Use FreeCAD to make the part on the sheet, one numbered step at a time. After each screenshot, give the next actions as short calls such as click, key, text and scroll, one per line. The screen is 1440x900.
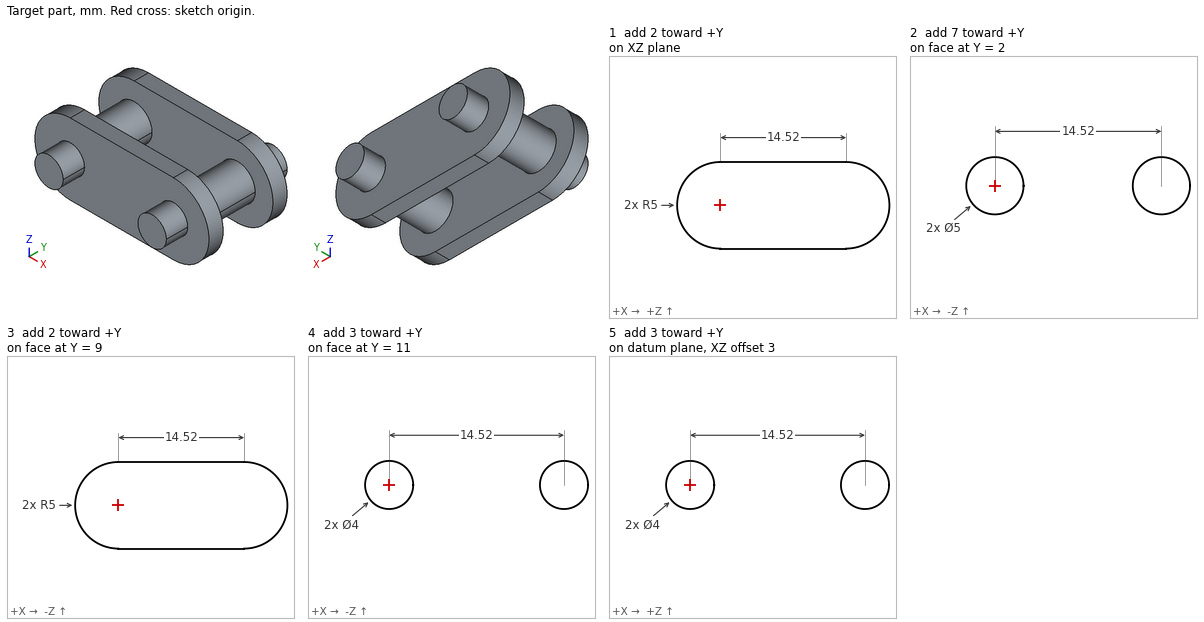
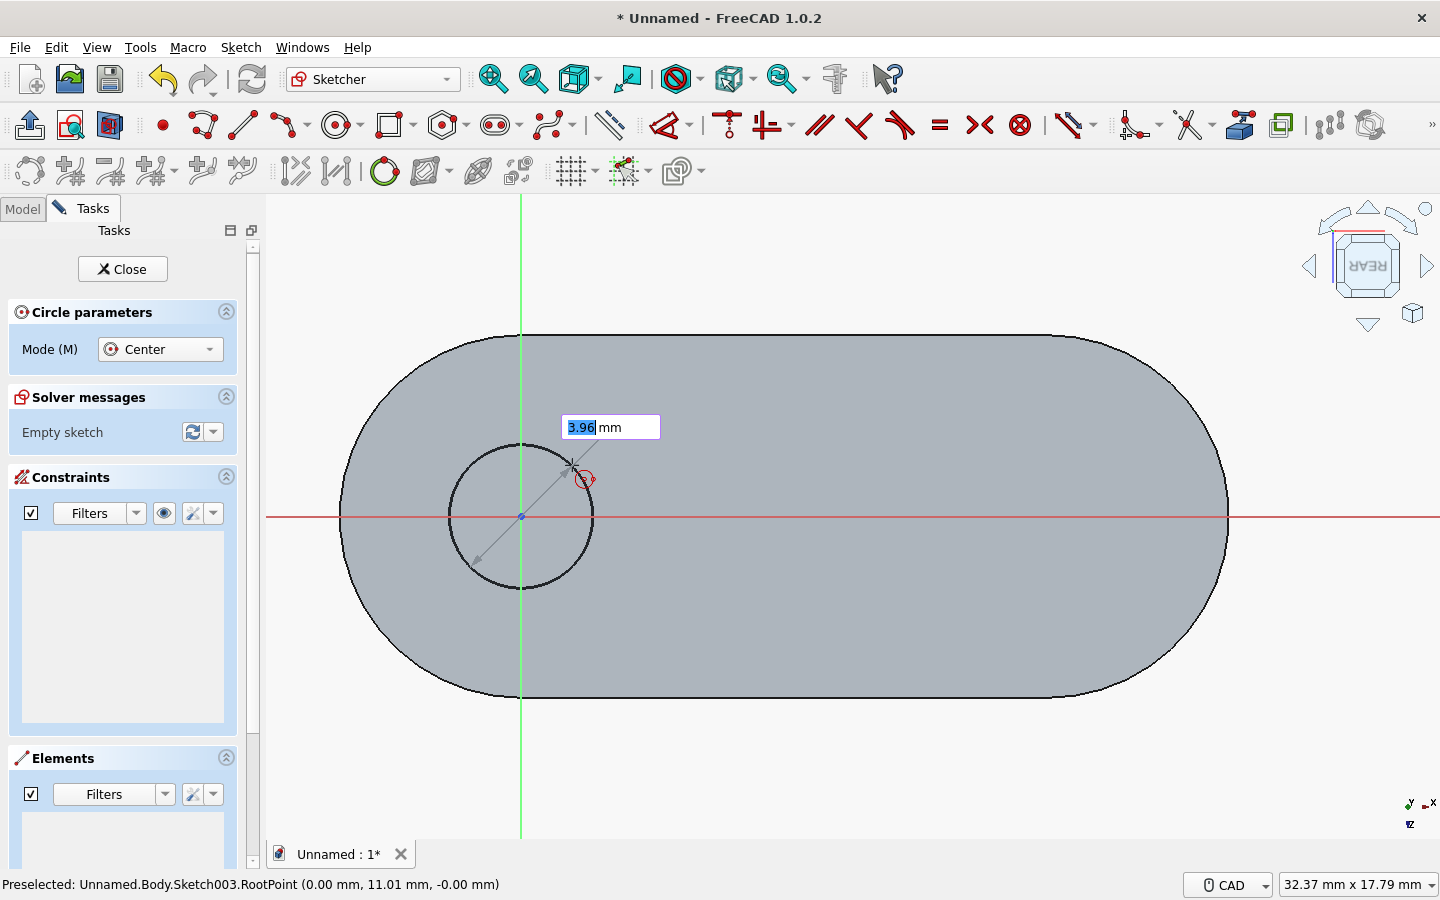
text(4)
key(Return)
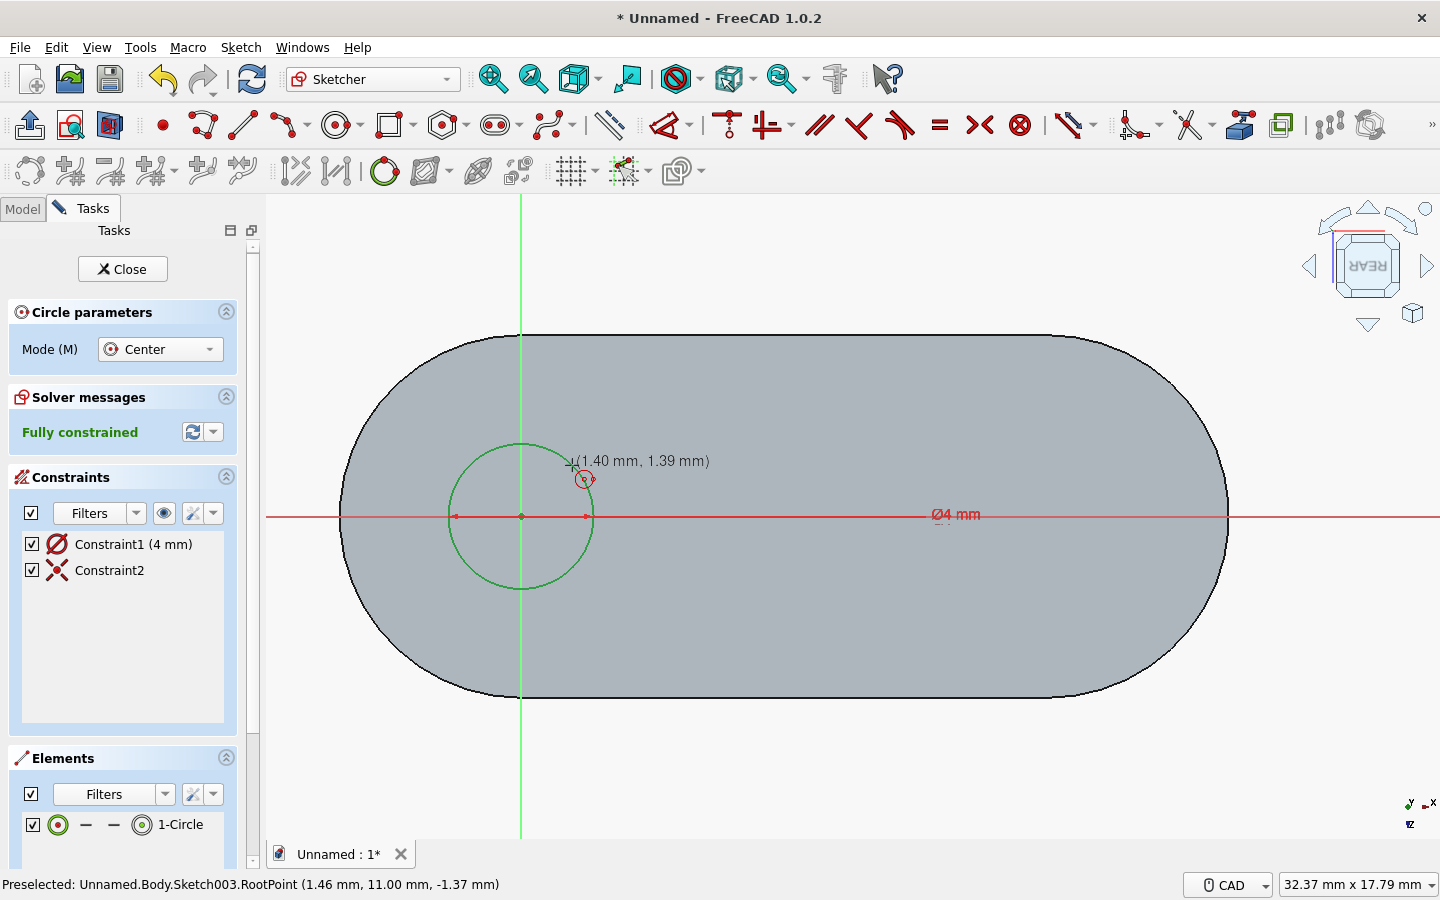
click(1048, 516)
move(1099, 465)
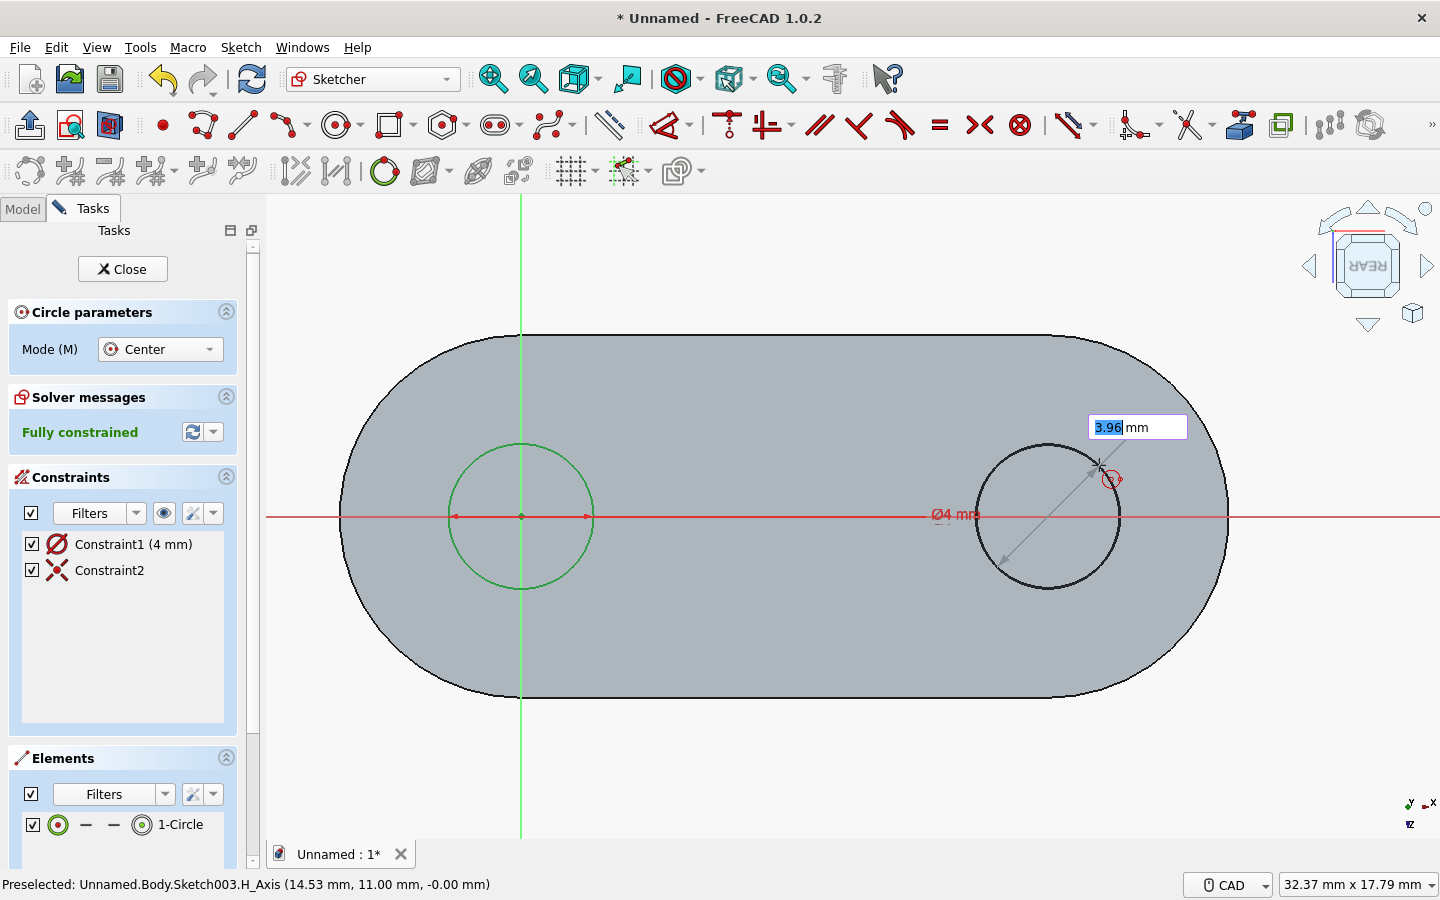
text(4)
key(Return)
key(Escape)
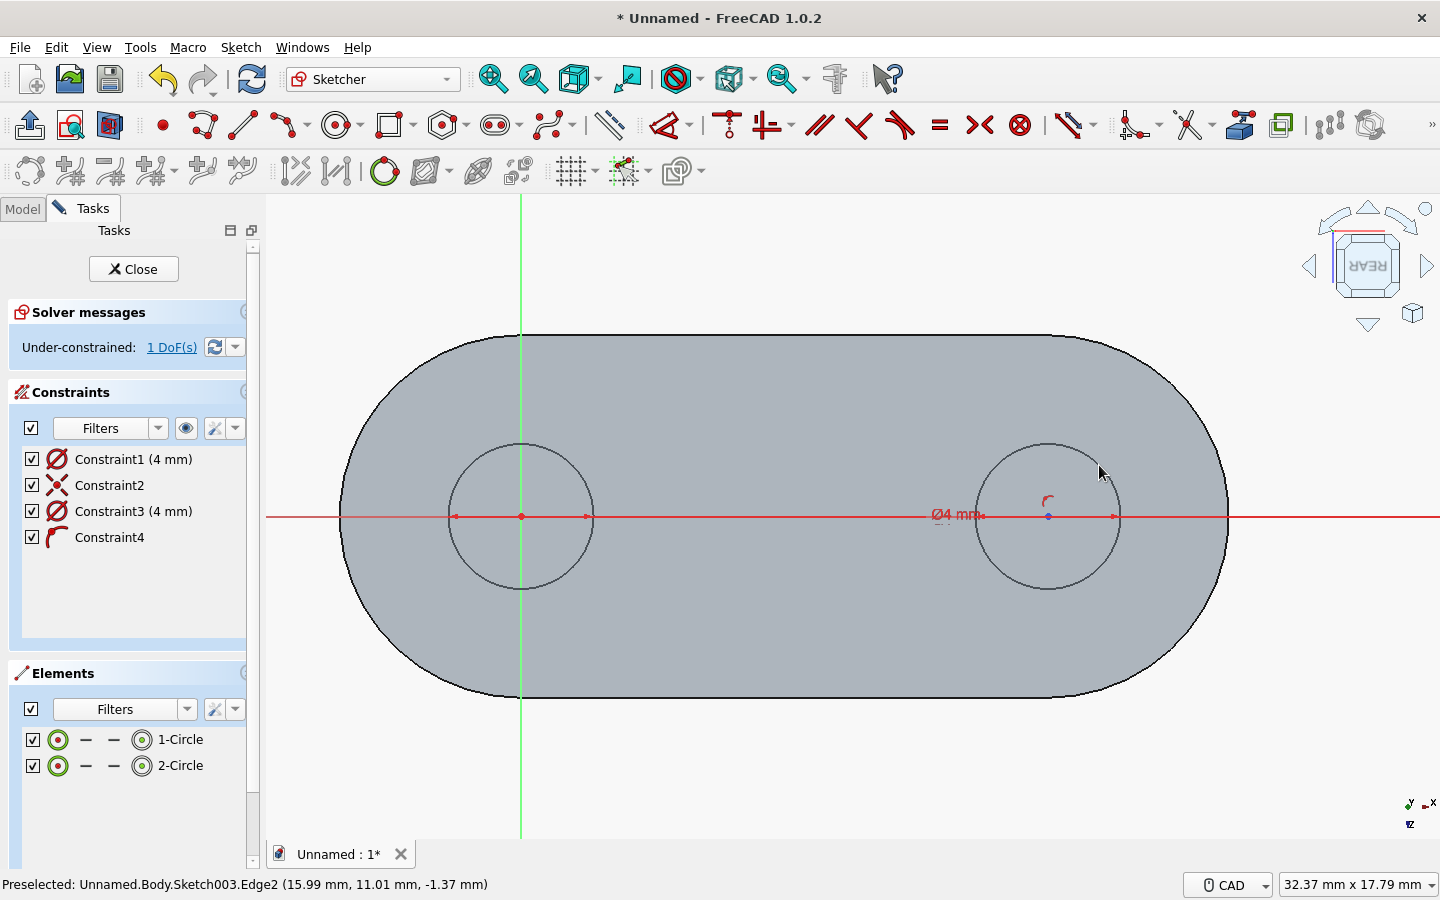
click(664, 126)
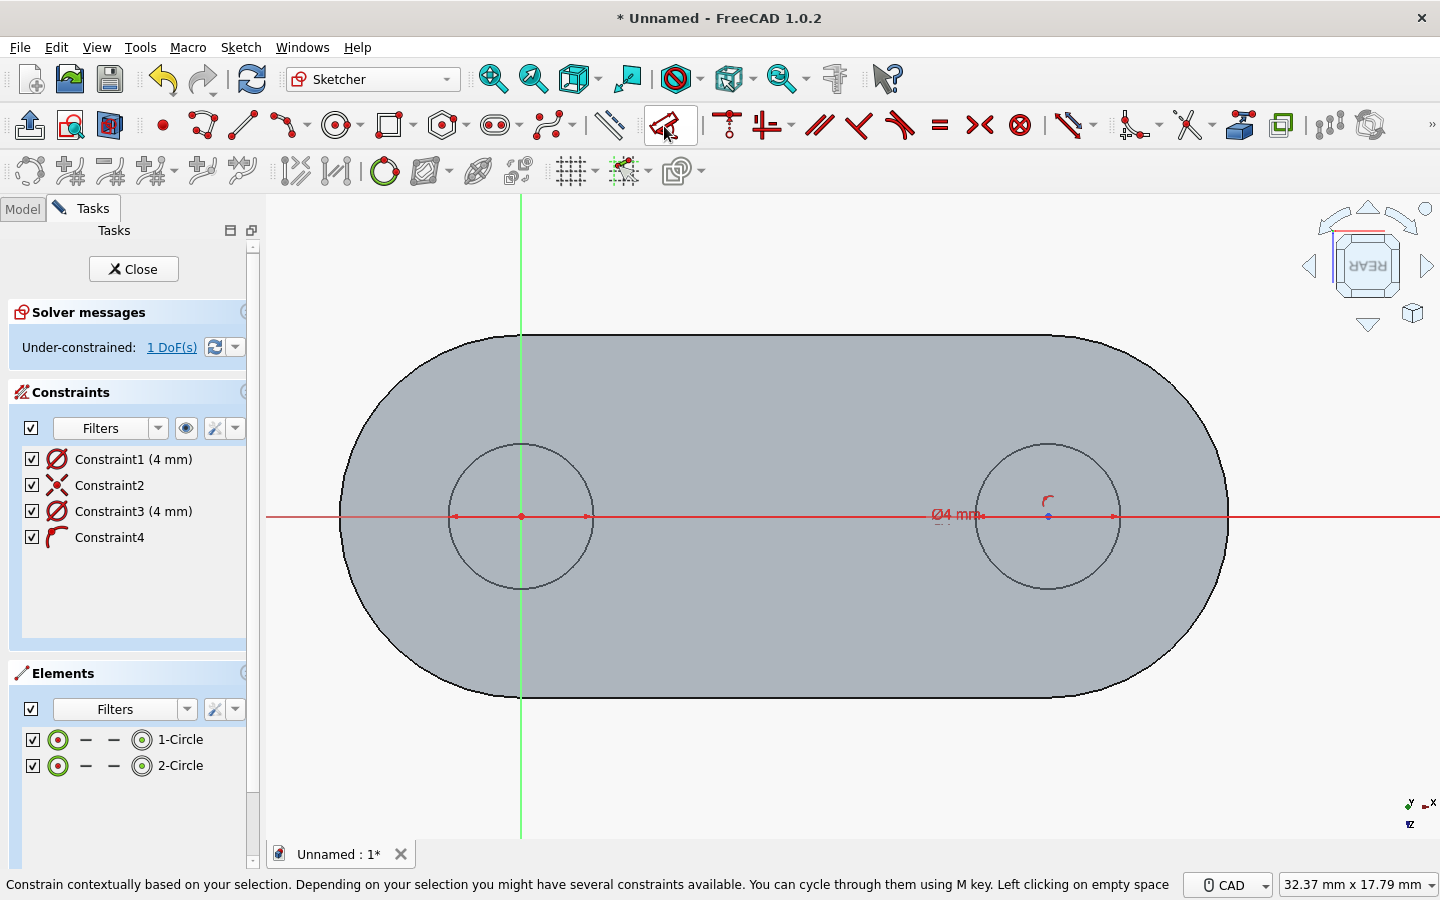
click(1048, 516)
click(785, 550)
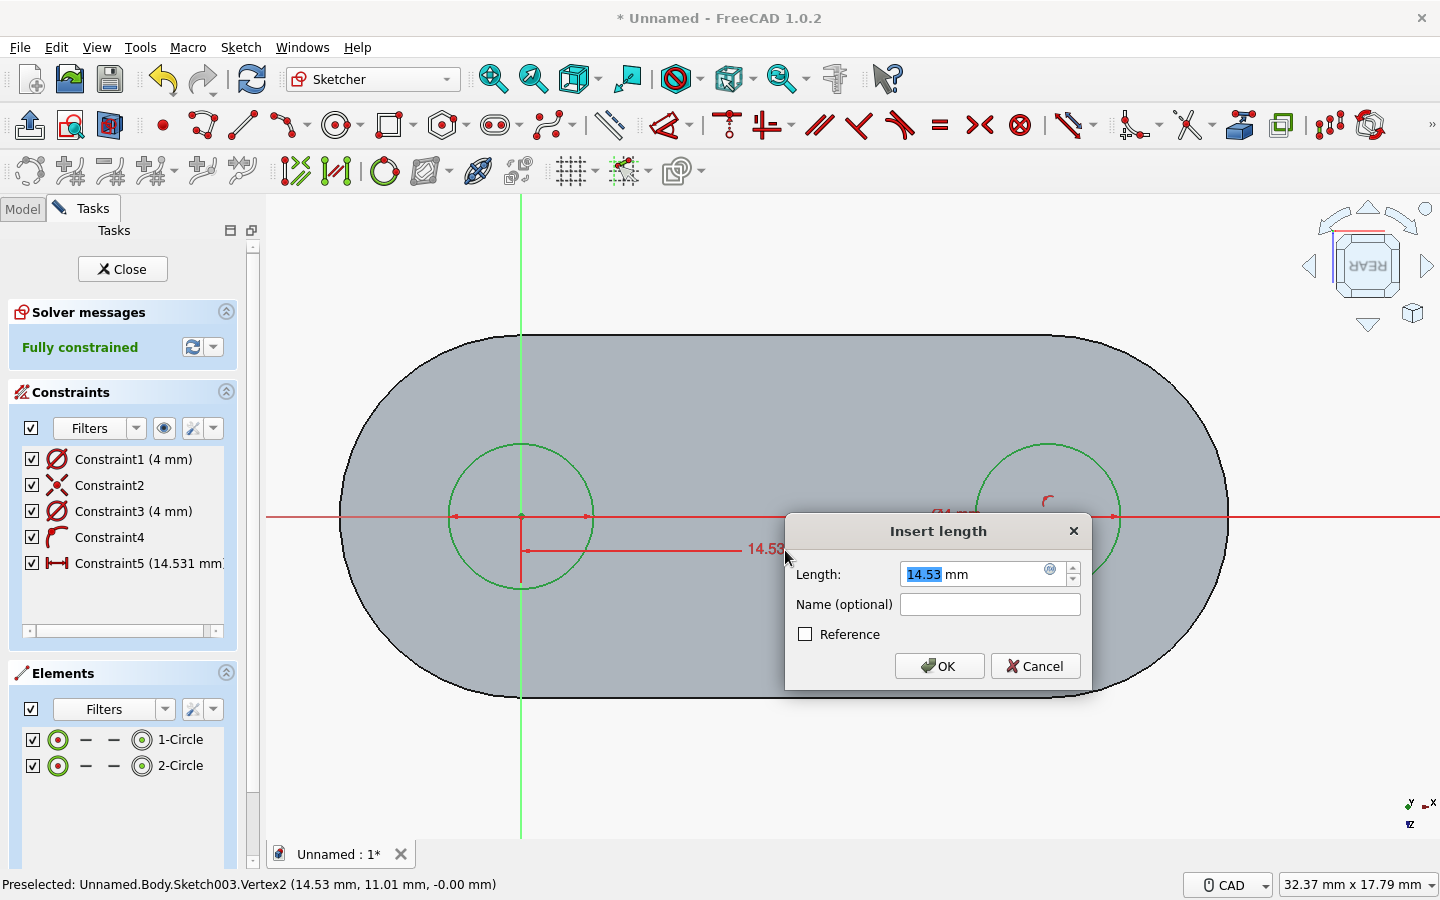
text(14.52)
key(Return)
key(Escape)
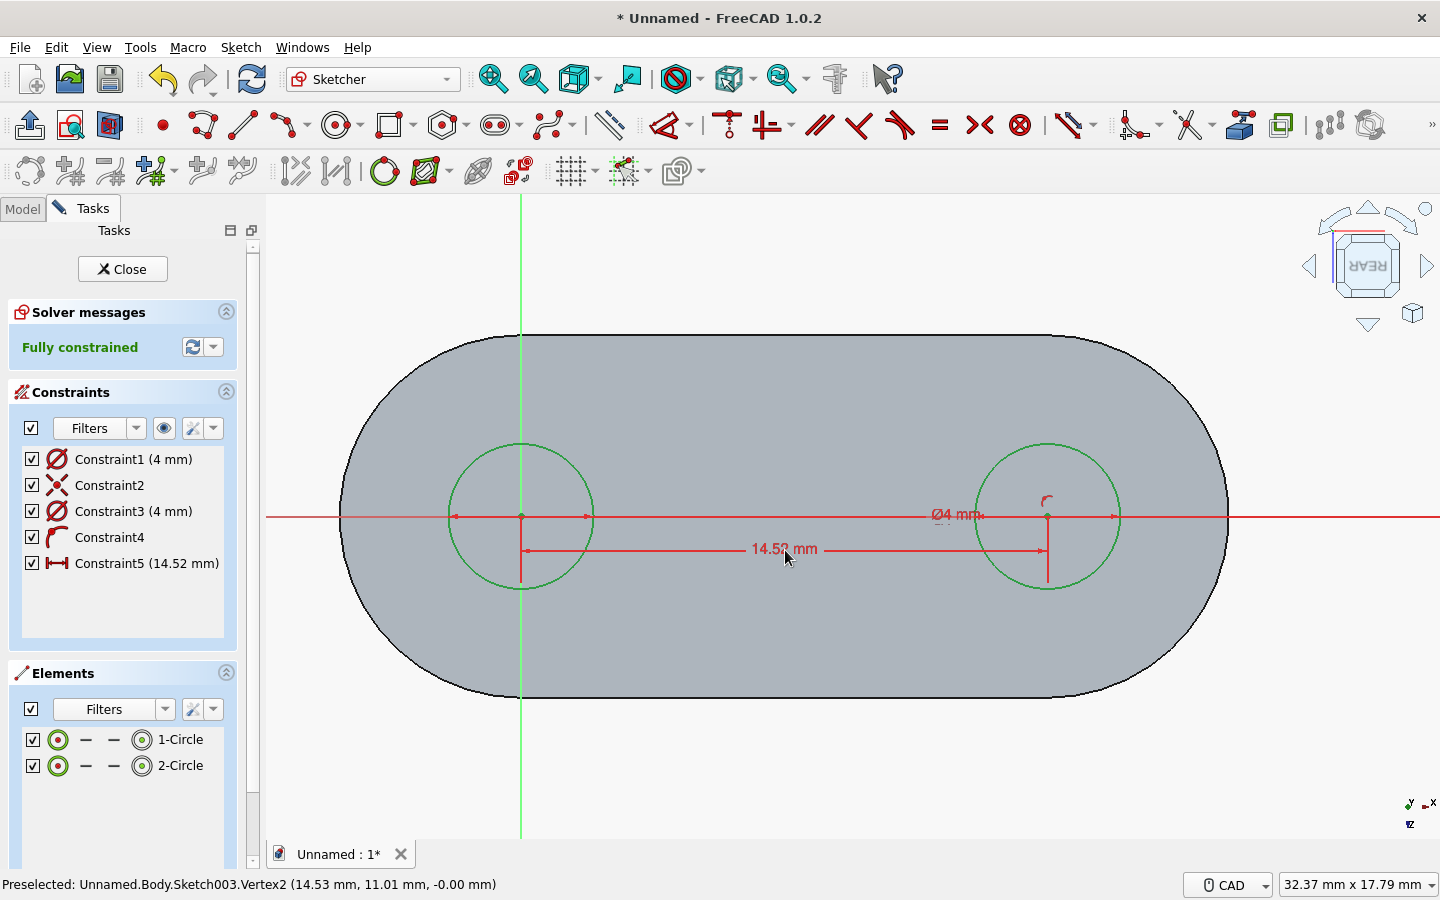
click(123, 269)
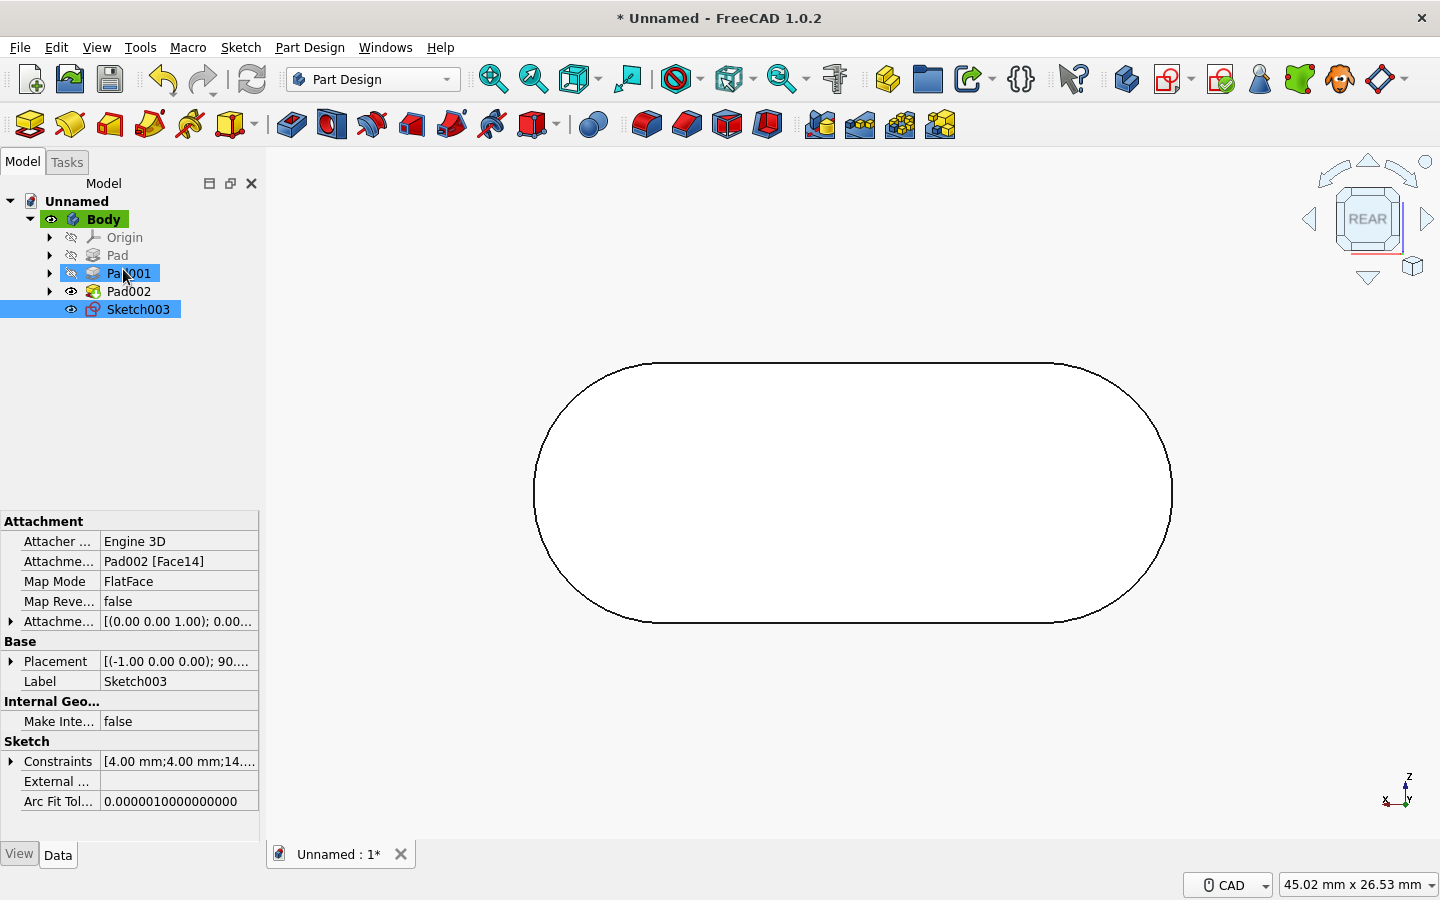
click(30, 124)